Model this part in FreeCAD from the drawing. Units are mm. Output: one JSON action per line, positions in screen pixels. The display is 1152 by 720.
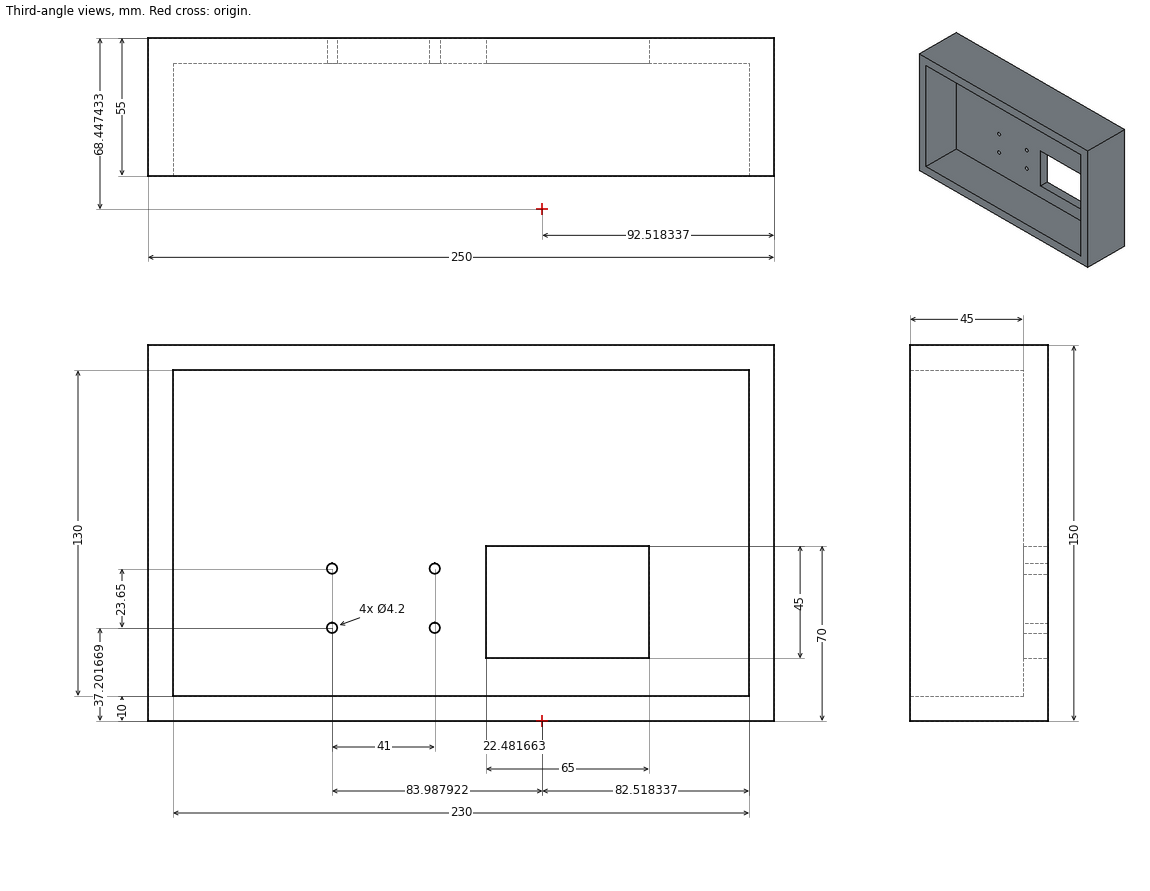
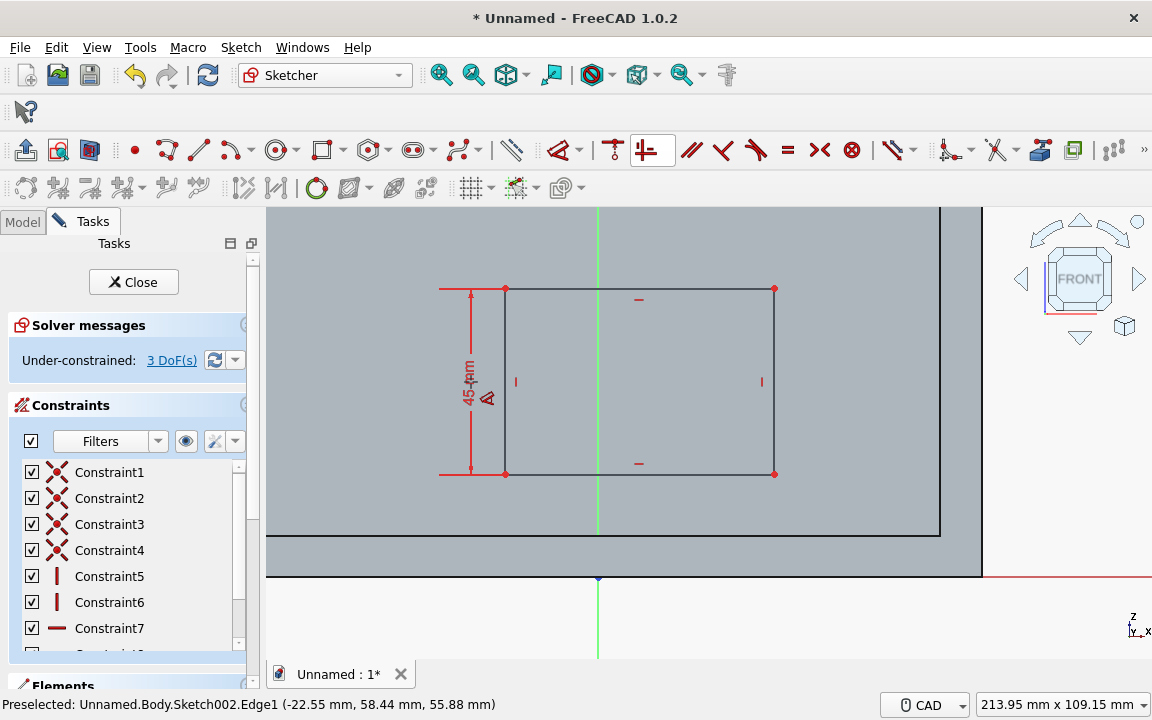
{"action": "left_click", "coordinate": [586, 475]}
{"action": "left_click", "coordinate": [639, 509]}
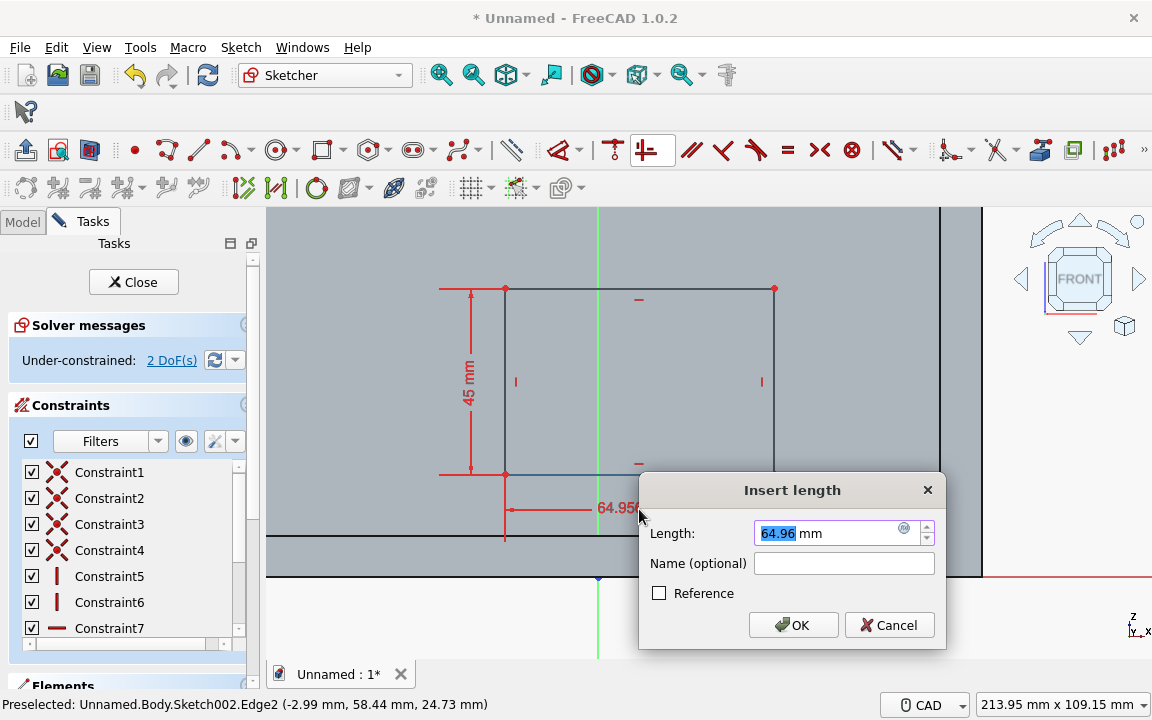
{"action": "type", "text": "65"}
{"action": "key", "text": "Return"}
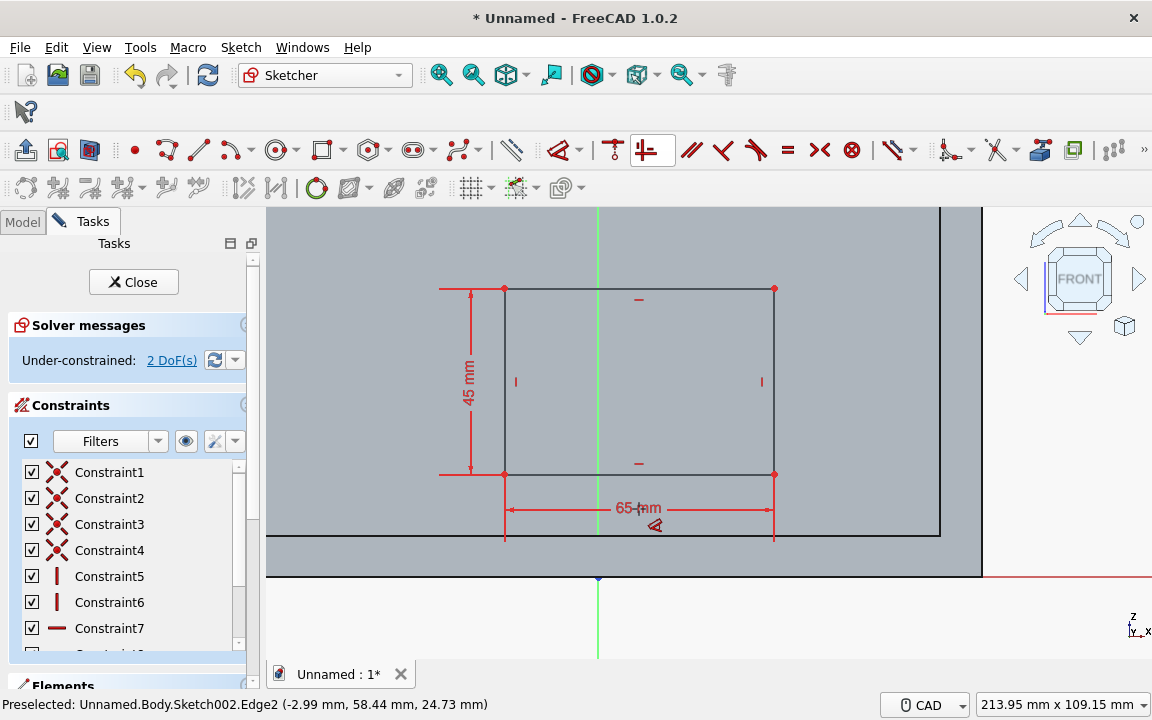
{"action": "left_click", "coordinate": [505, 289]}
{"action": "left_click", "coordinate": [471, 433]}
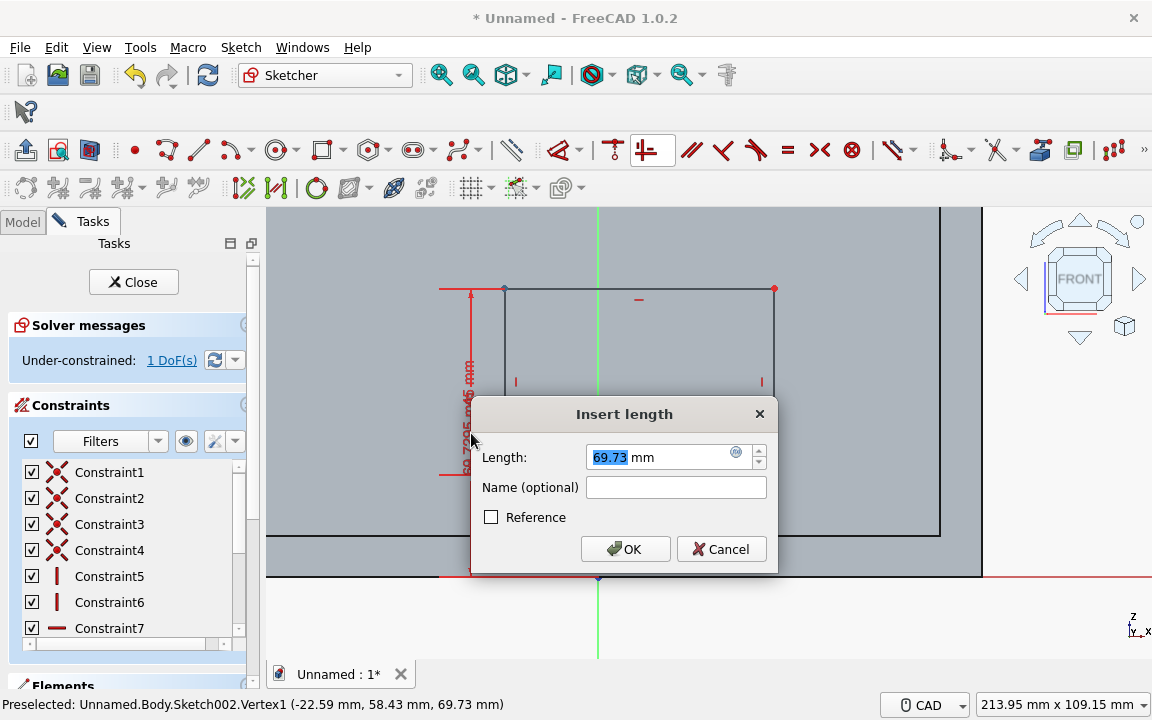
{"action": "type", "text": "70"}
{"action": "key", "text": "Return"}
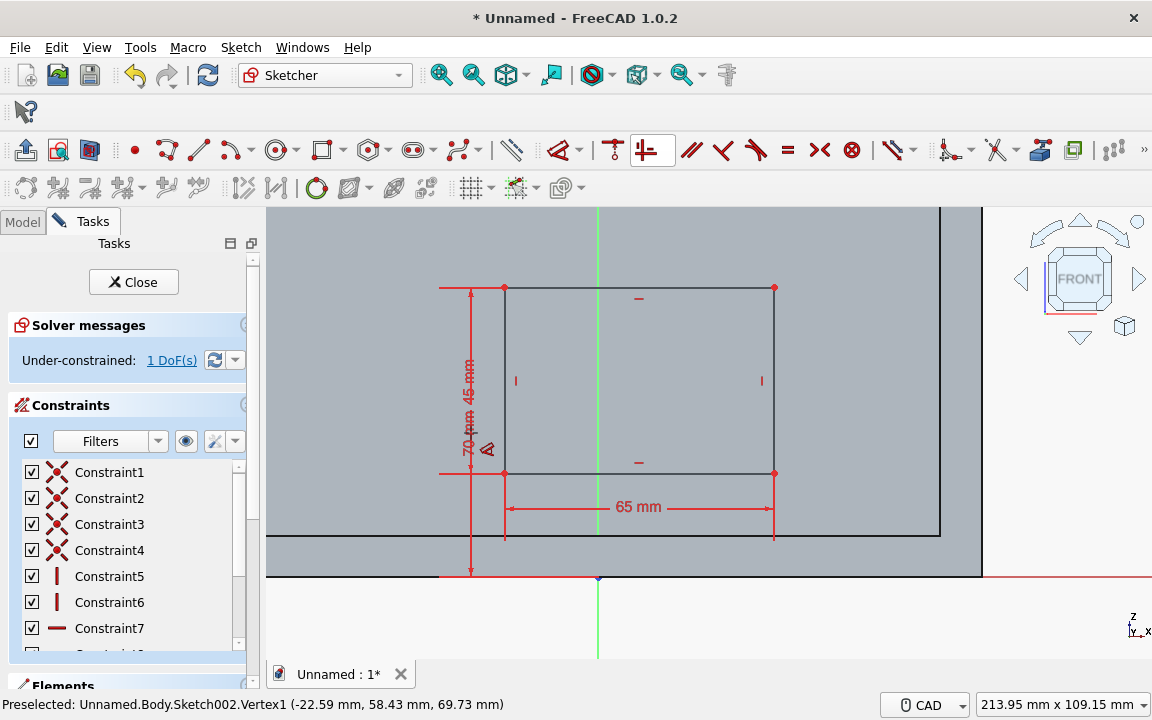
{"action": "left_click", "coordinate": [505, 288]}
{"action": "left_click", "coordinate": [552, 611]}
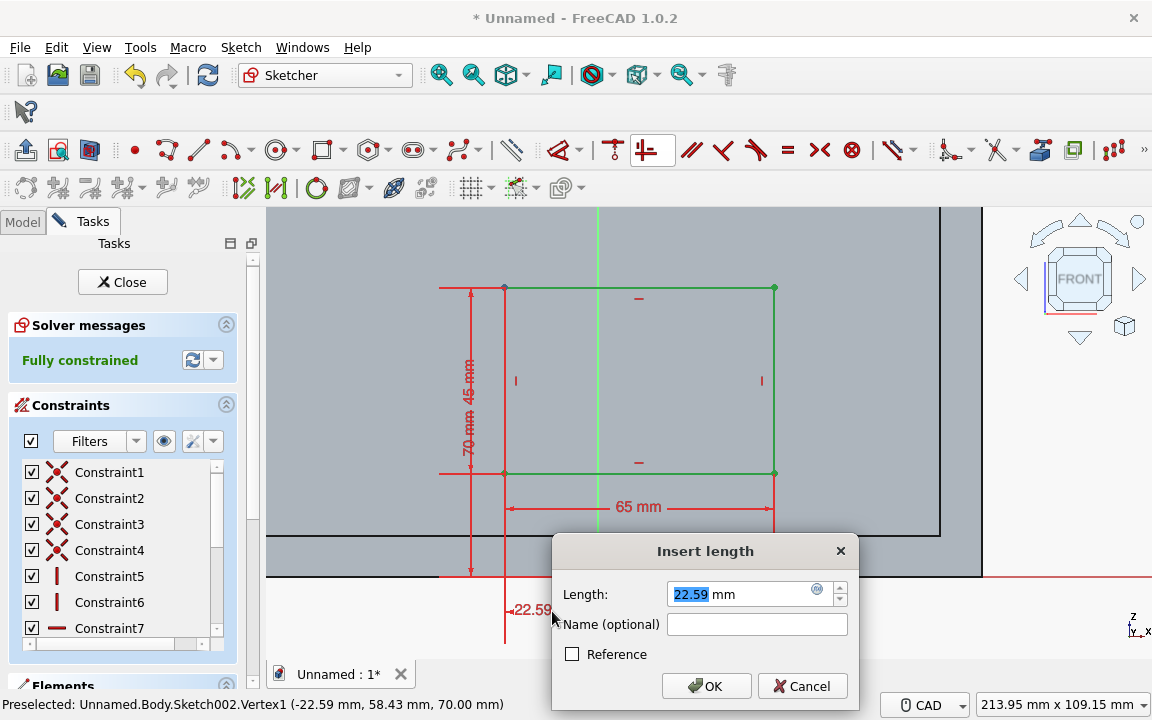
{"action": "type", "text": "22.481663"}
{"action": "key", "text": "Return"}
{"action": "key", "text": "Escape"}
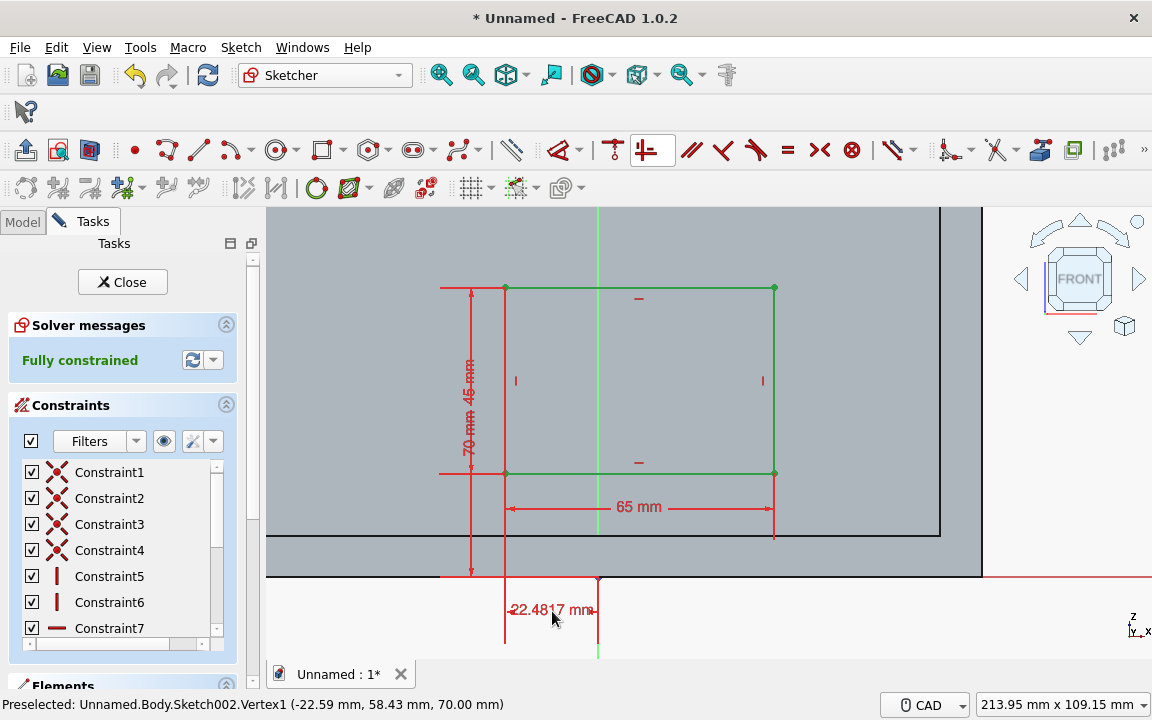
{"action": "left_click", "coordinate": [123, 282]}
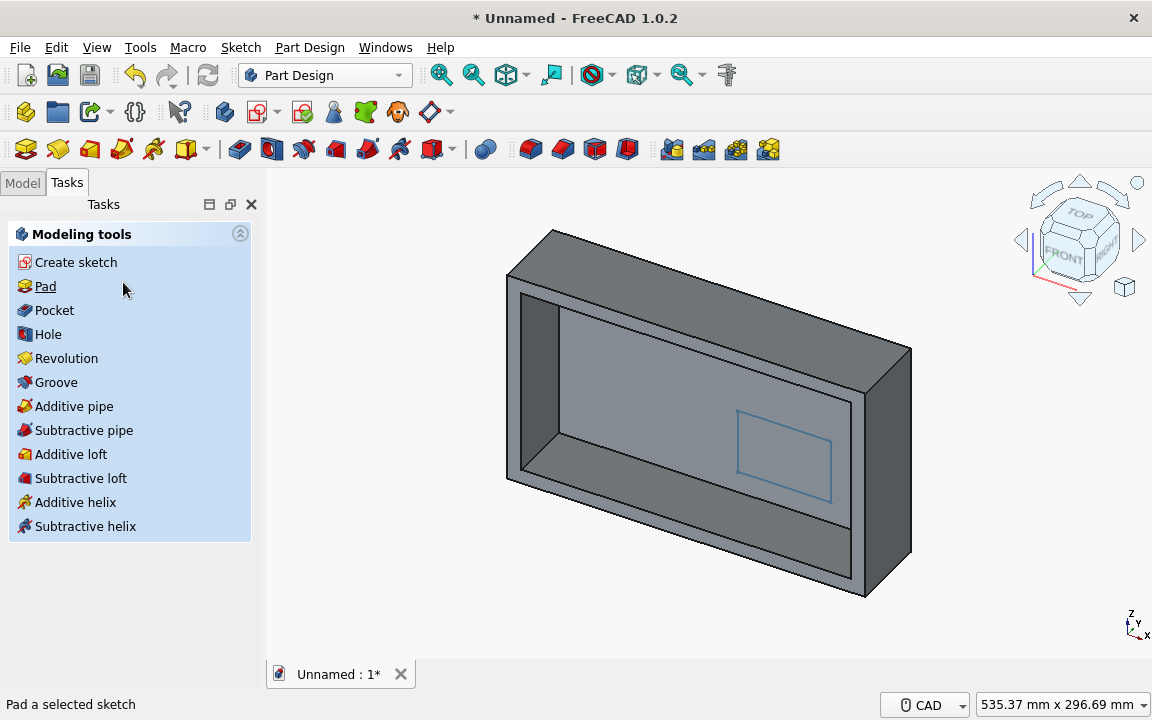
{"action": "left_click", "coordinate": [240, 150]}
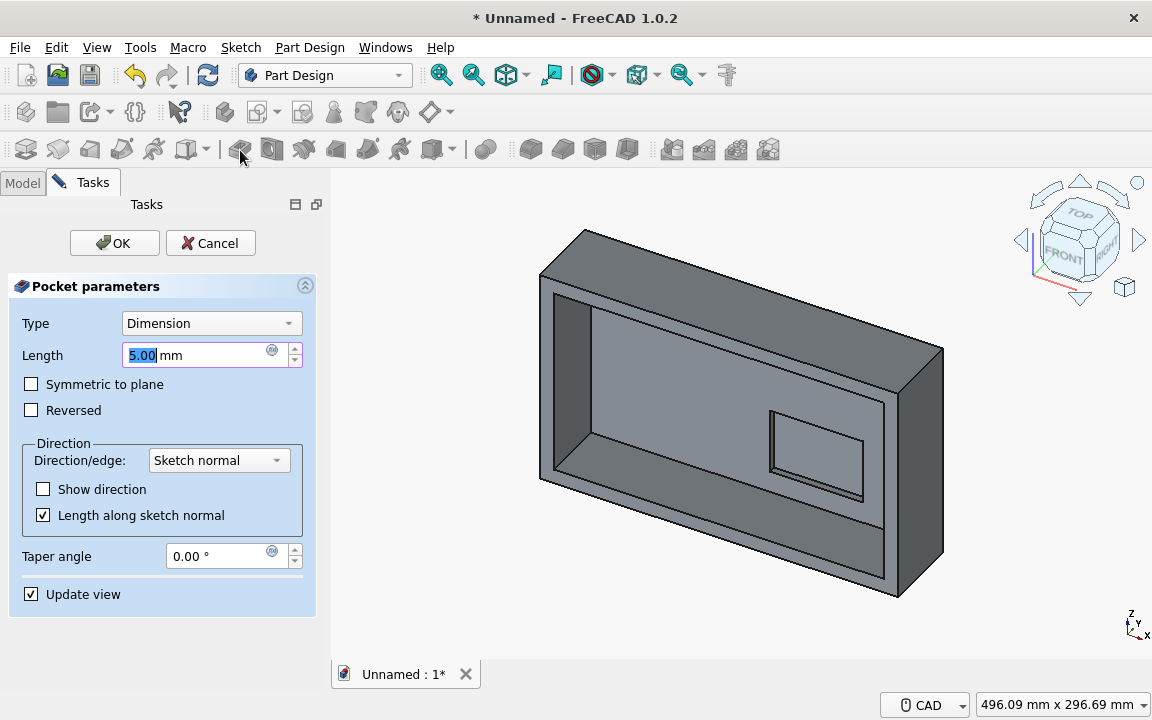
{"action": "left_click", "coordinate": [212, 324]}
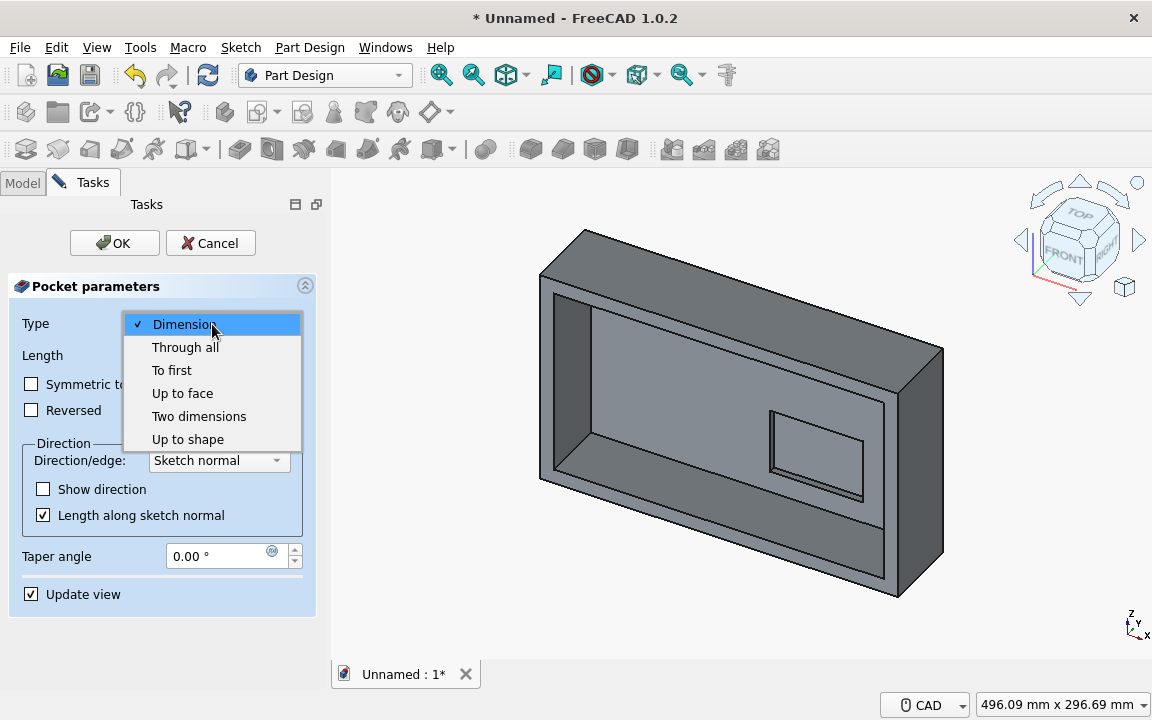
{"action": "left_click", "coordinate": [212, 348]}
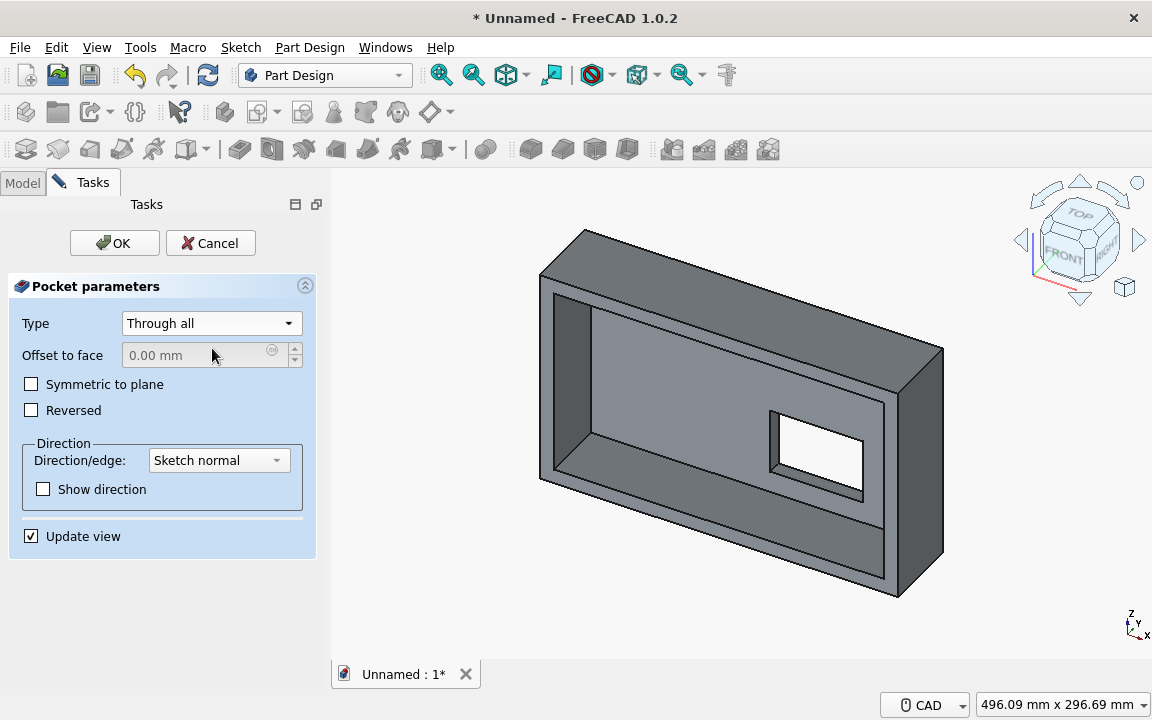
{"action": "left_click", "coordinate": [115, 243]}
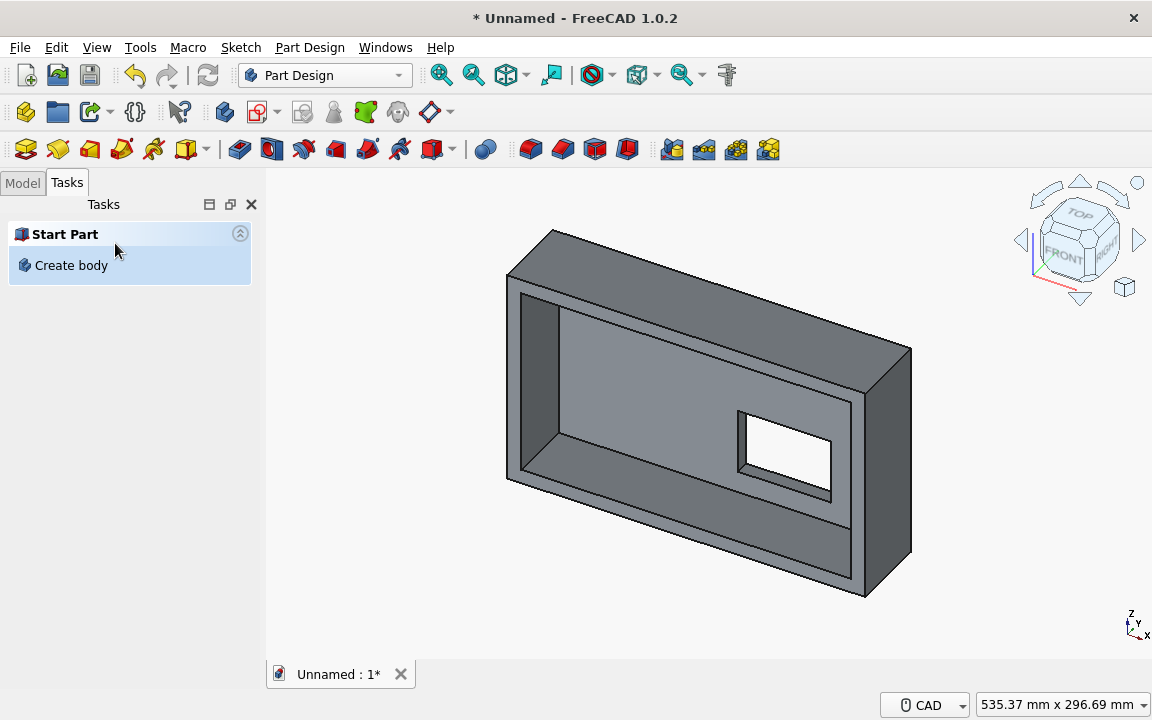
{"action": "left_click", "coordinate": [23, 182]}